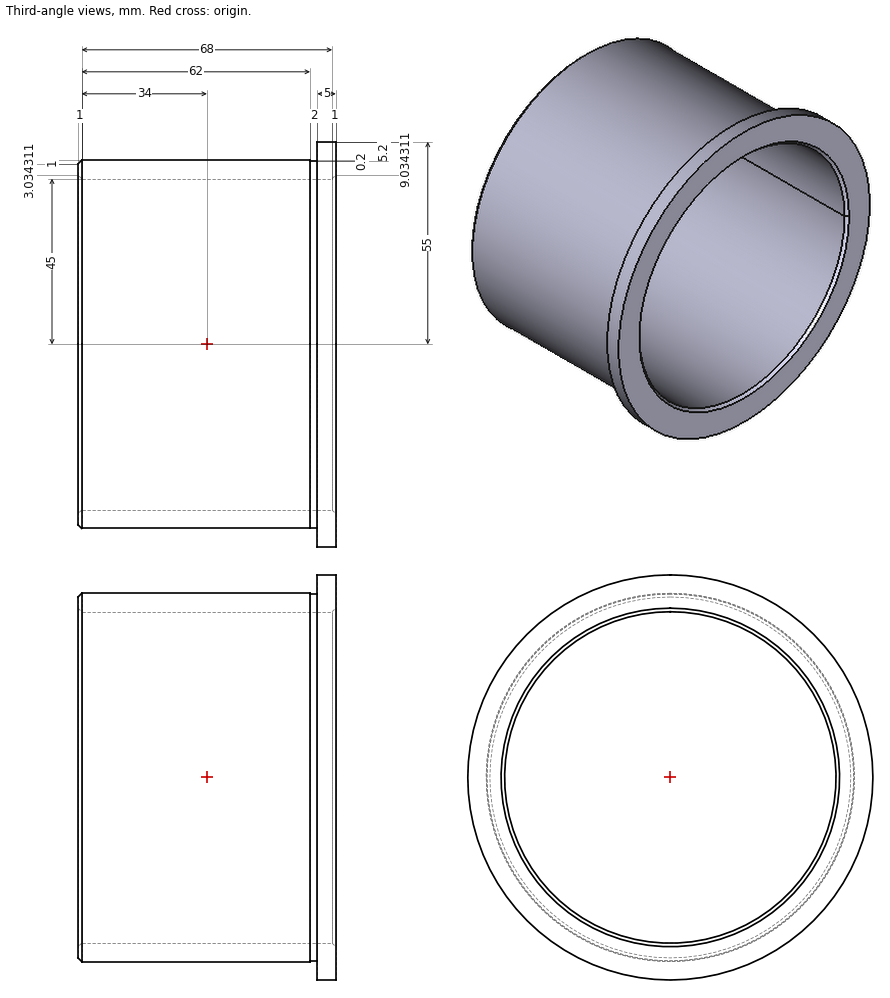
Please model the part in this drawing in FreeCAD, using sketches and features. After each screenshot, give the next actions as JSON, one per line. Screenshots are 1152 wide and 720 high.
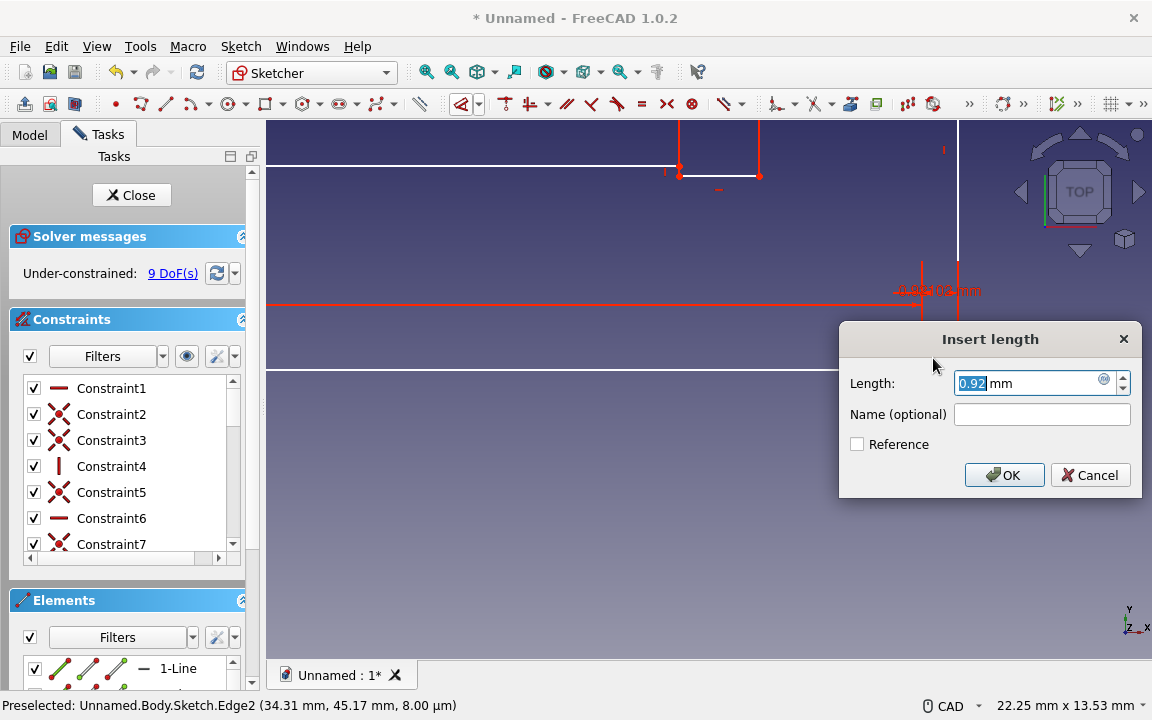
{"action": "type", "text": "1"}
{"action": "key", "text": "Return"}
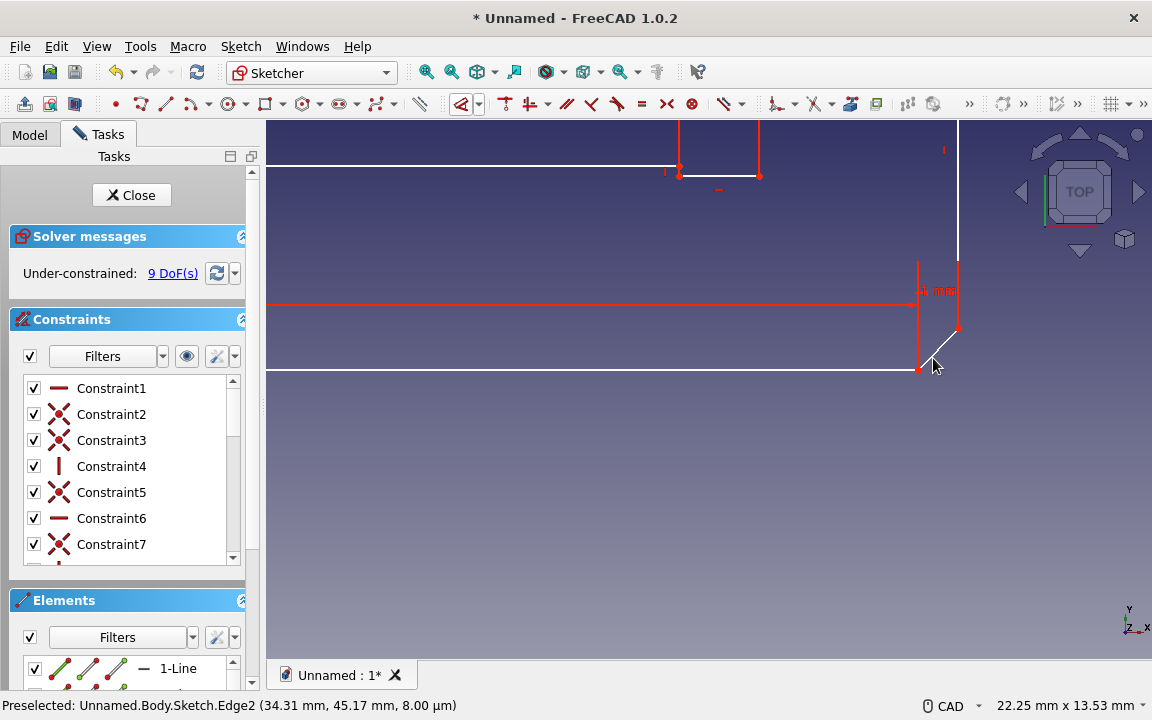
{"action": "scroll", "coordinate": [853, 256], "scroll_direction": "down", "scroll_amount": 9}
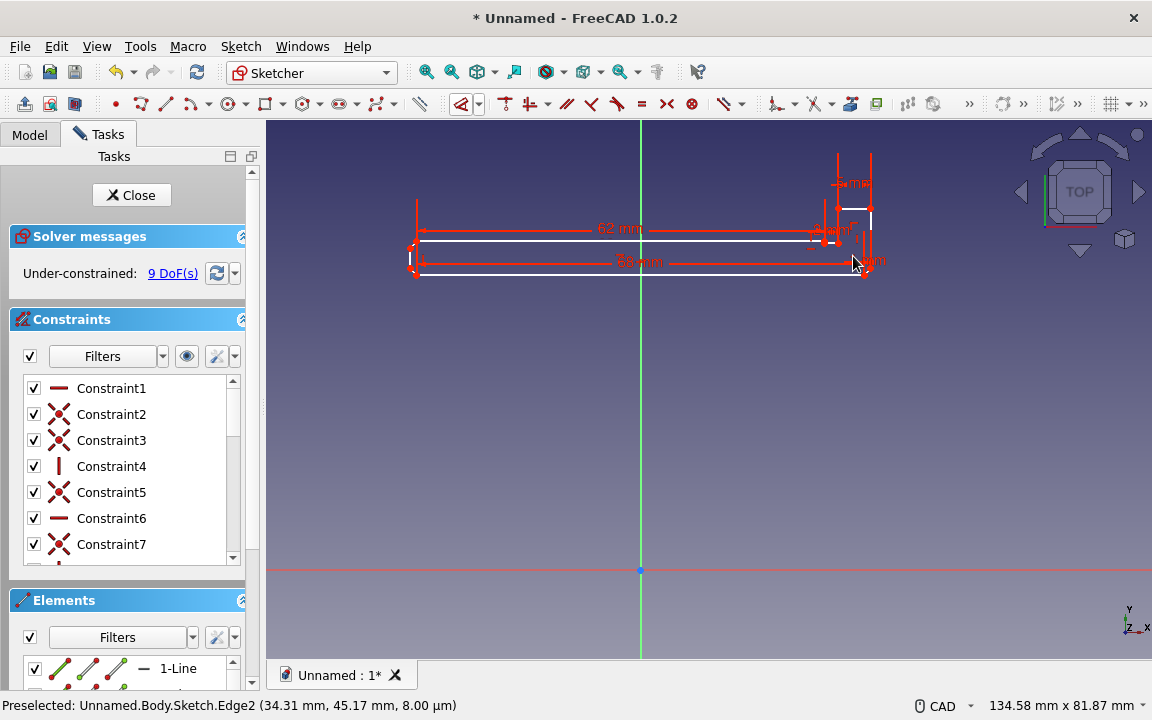
{"action": "scroll", "coordinate": [415, 244], "scroll_direction": "up", "scroll_amount": 9}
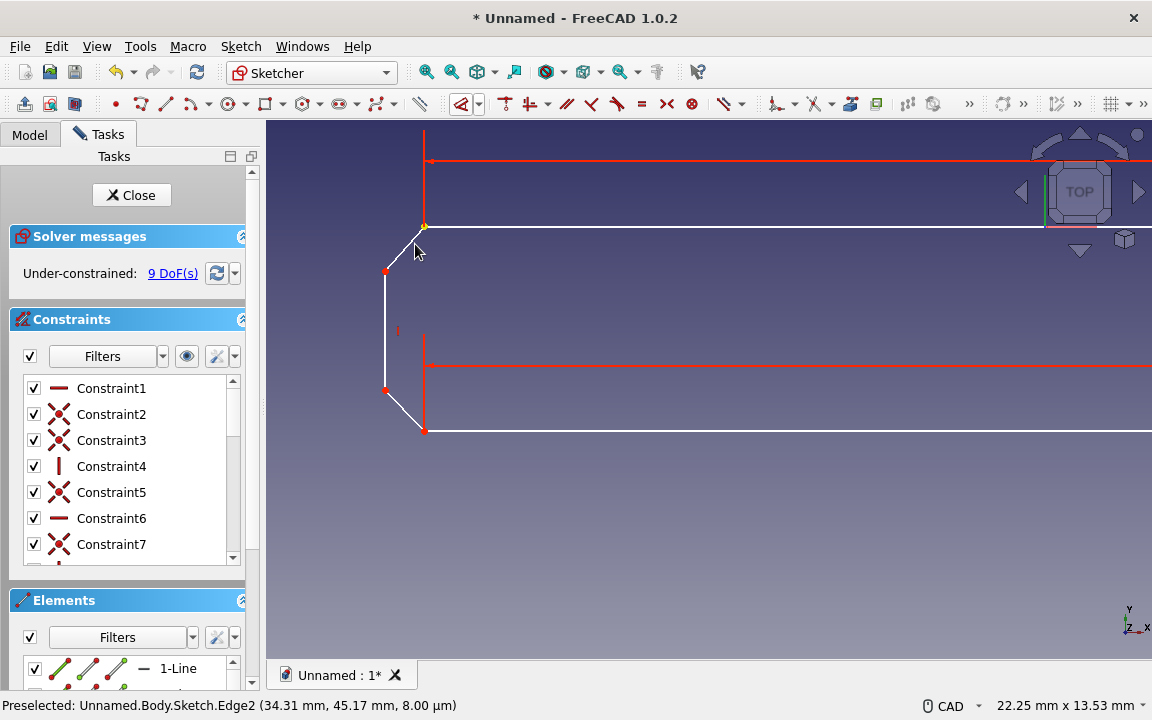
{"action": "left_click", "coordinate": [413, 240]}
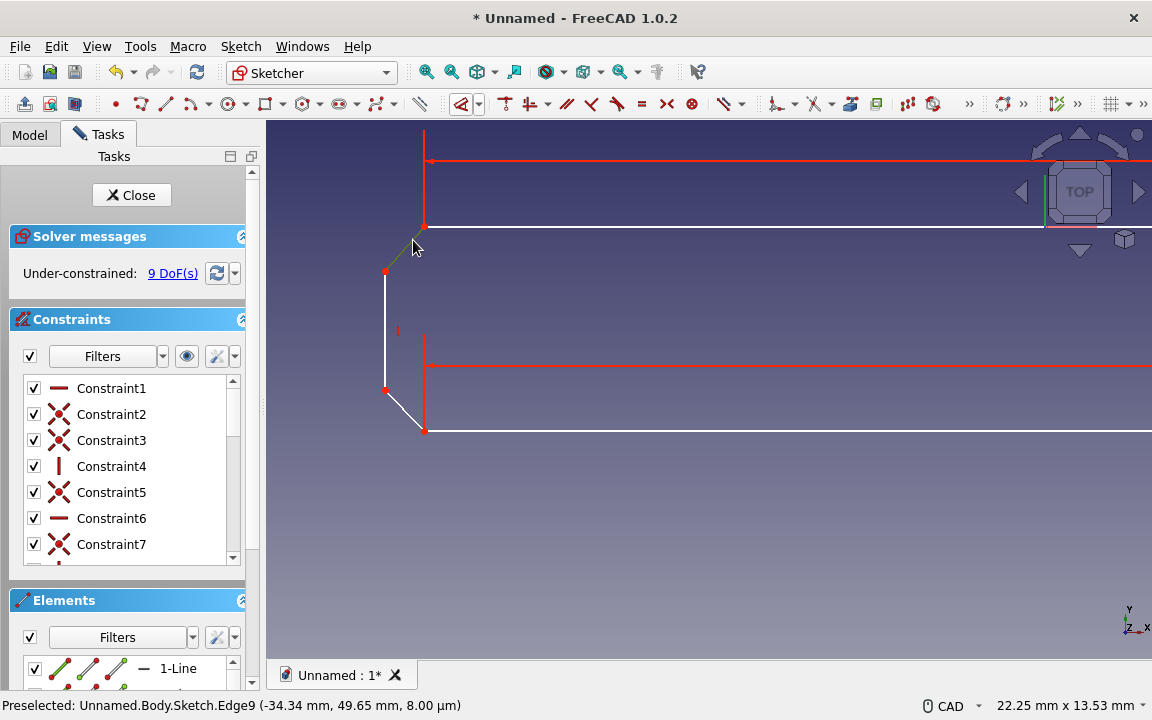
{"action": "left_click", "coordinate": [478, 104]}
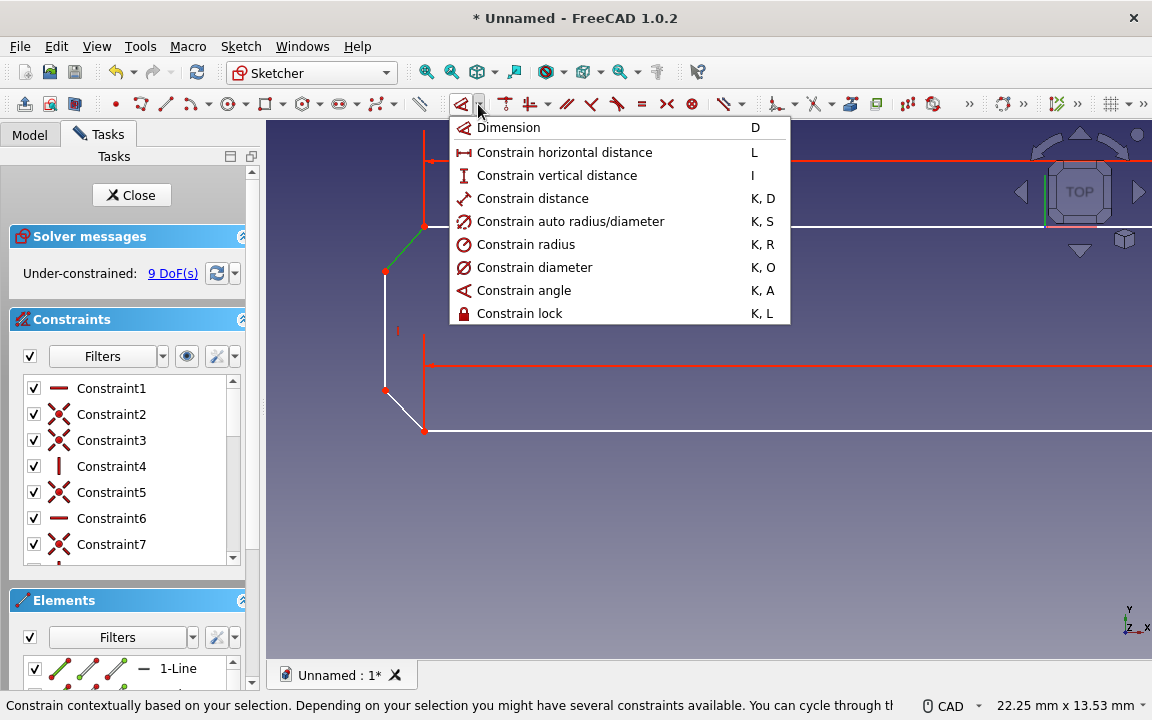
{"action": "left_click", "coordinate": [620, 152]}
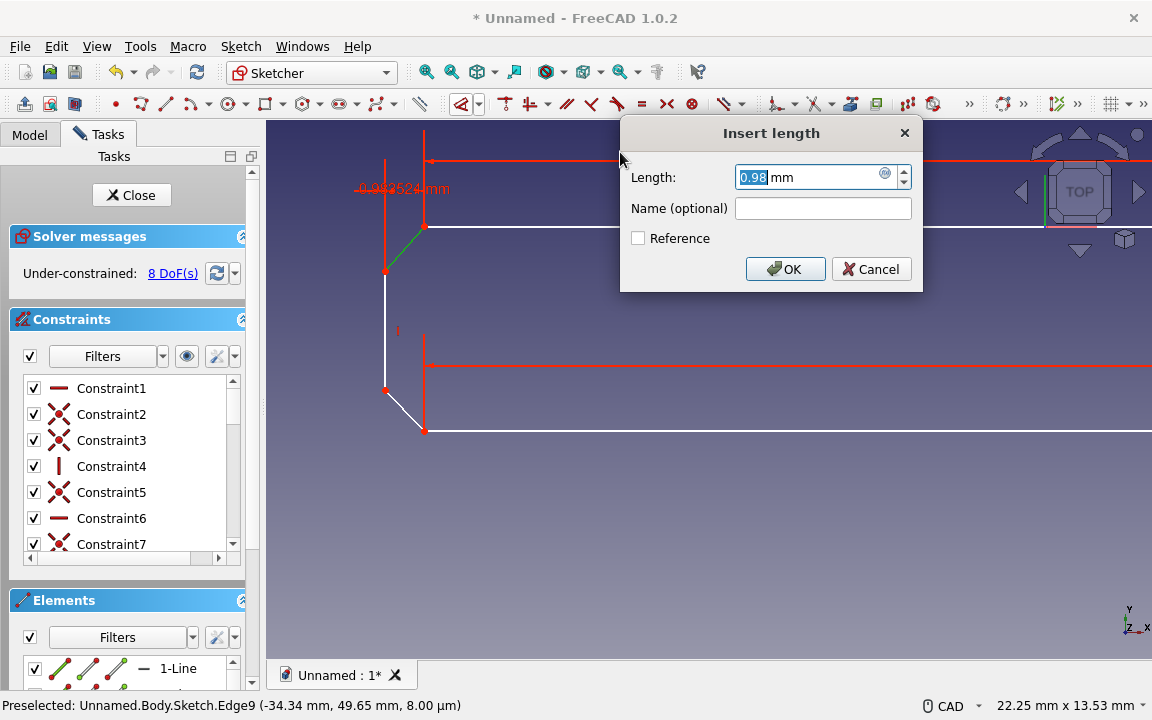
{"action": "type", "text": "1"}
{"action": "key", "text": "Return"}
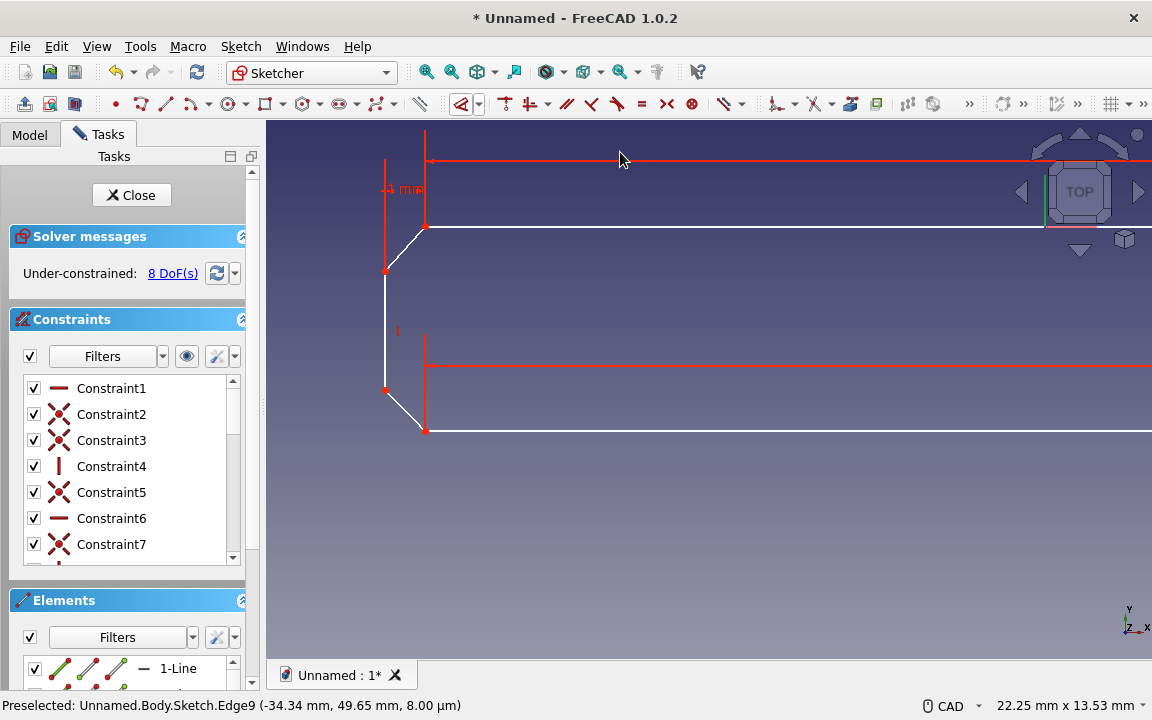
{"action": "left_click", "coordinate": [413, 240]}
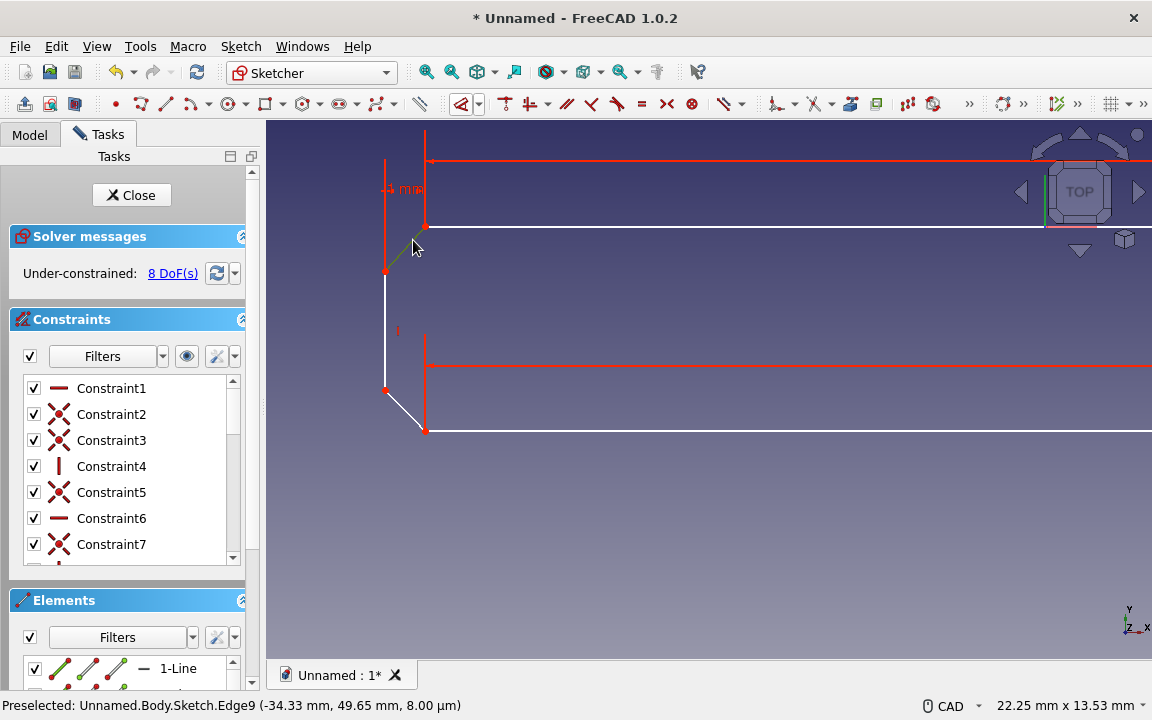
{"action": "key", "text": "i"}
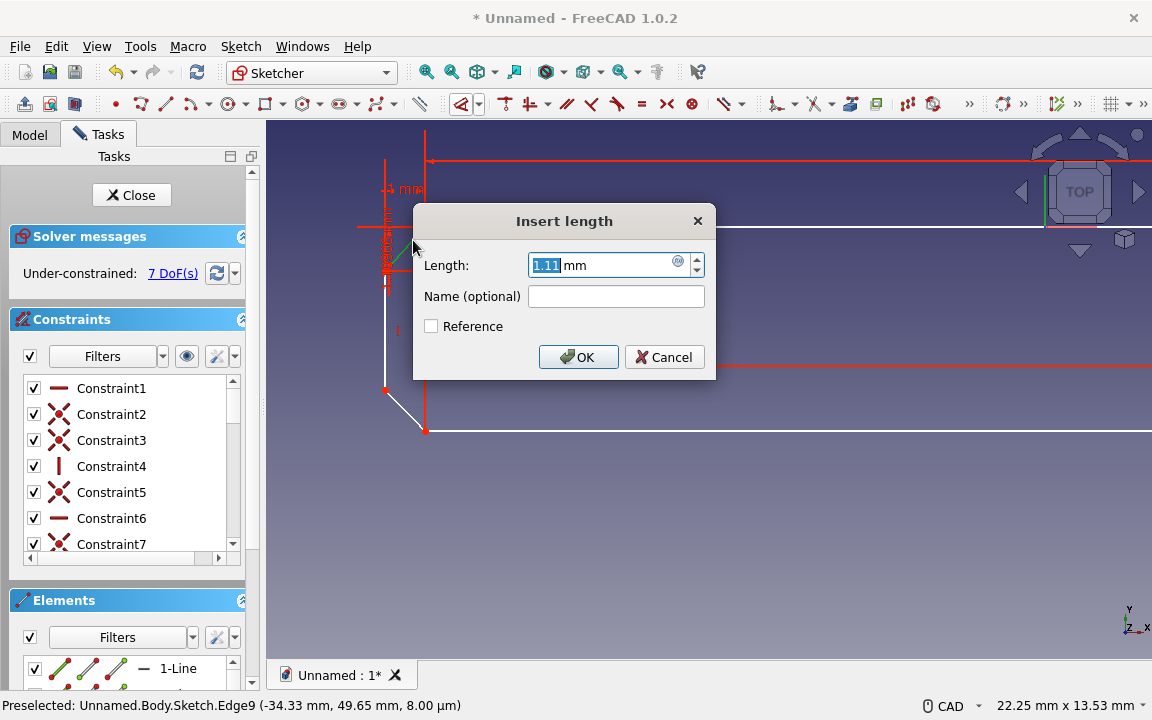
{"action": "type", "text": "1"}
{"action": "key", "text": "Return"}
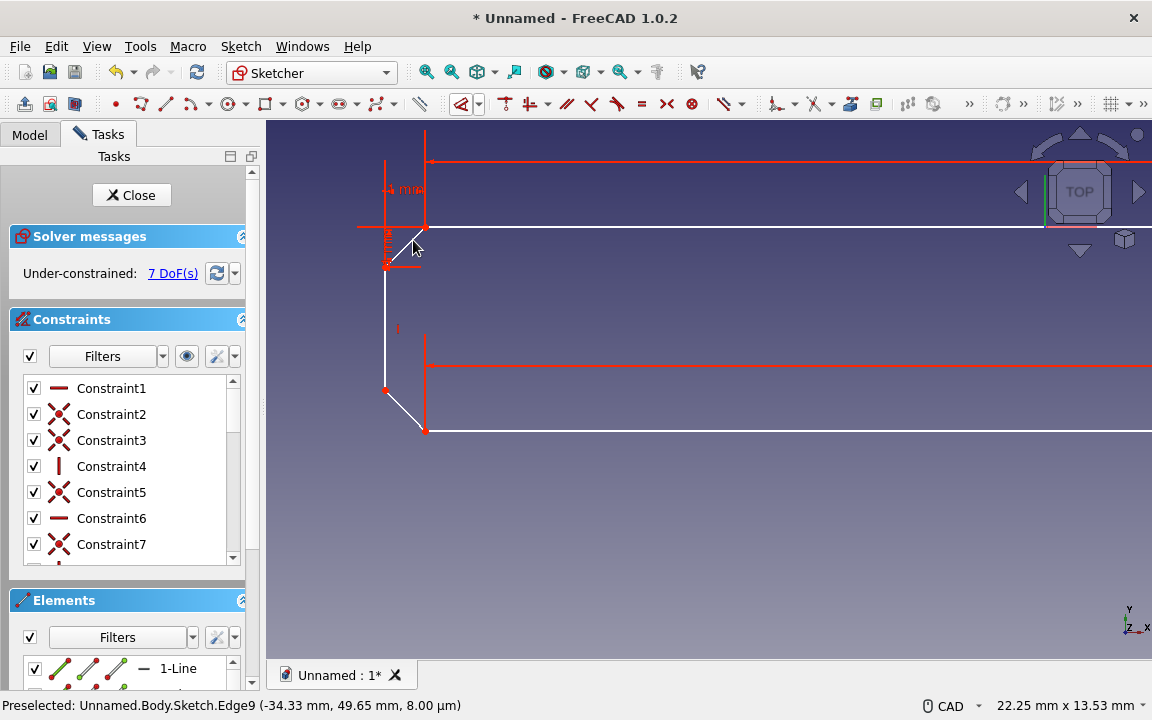
{"action": "scroll", "coordinate": [415, 244], "scroll_direction": "down", "scroll_amount": 9}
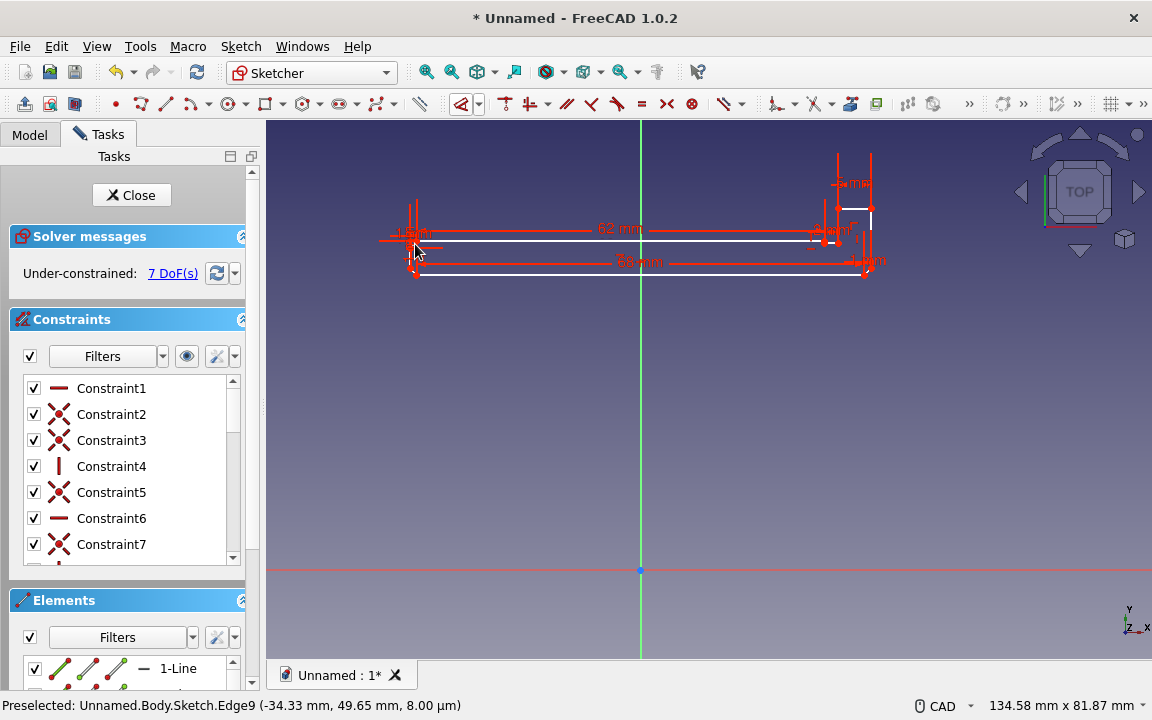
{"action": "scroll", "coordinate": [838, 219], "scroll_direction": "up", "scroll_amount": 2}